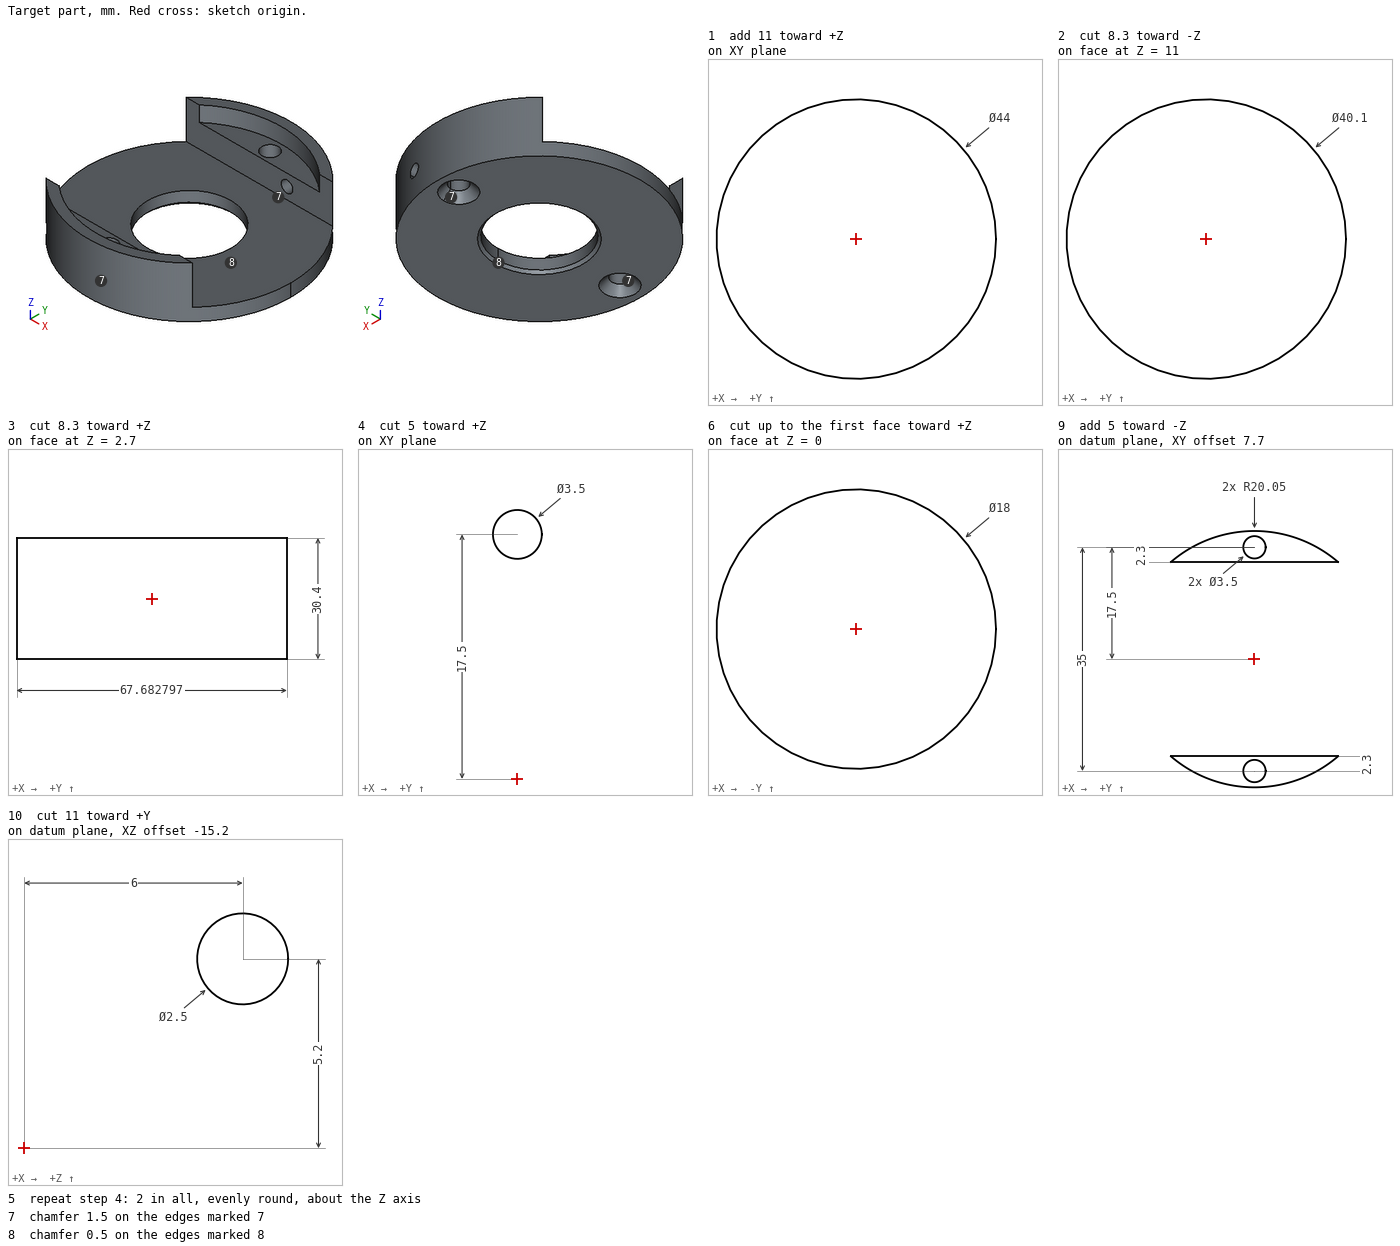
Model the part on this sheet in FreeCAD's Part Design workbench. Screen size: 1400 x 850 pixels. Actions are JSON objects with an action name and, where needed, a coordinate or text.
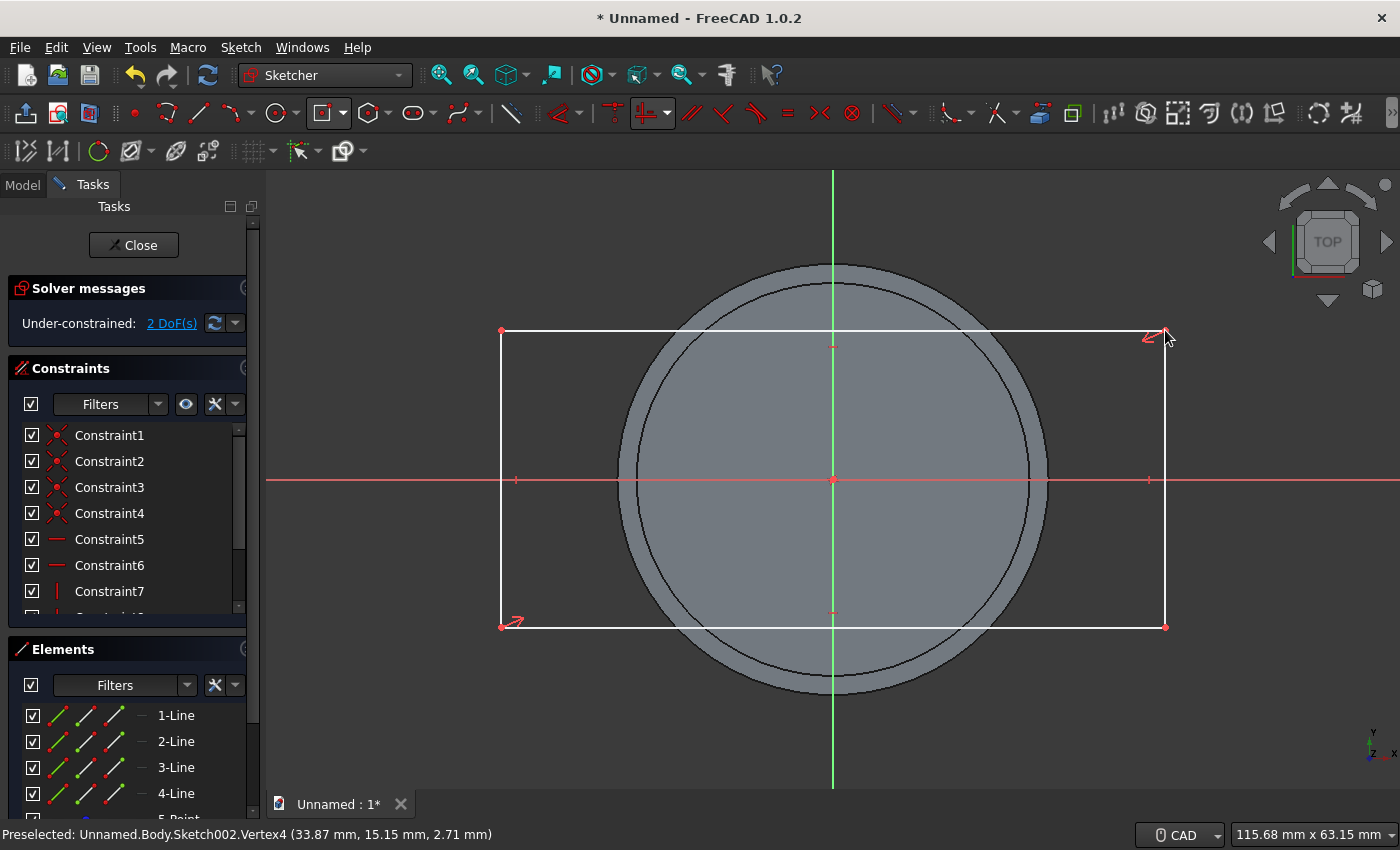
{"action": "left_click", "coordinate": [558, 114]}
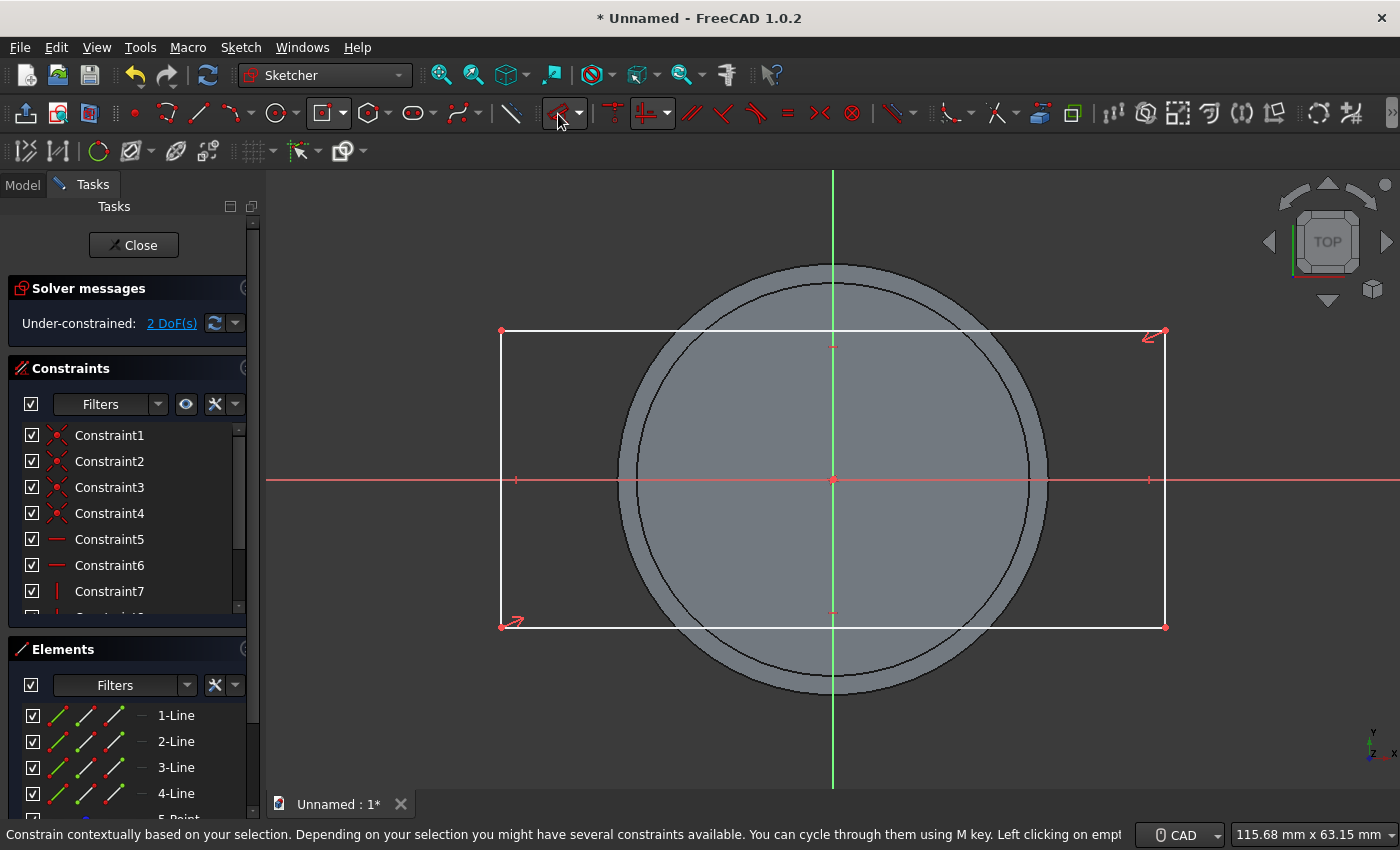
{"action": "left_click", "coordinate": [1165, 539]}
{"action": "left_click", "coordinate": [1199, 411]}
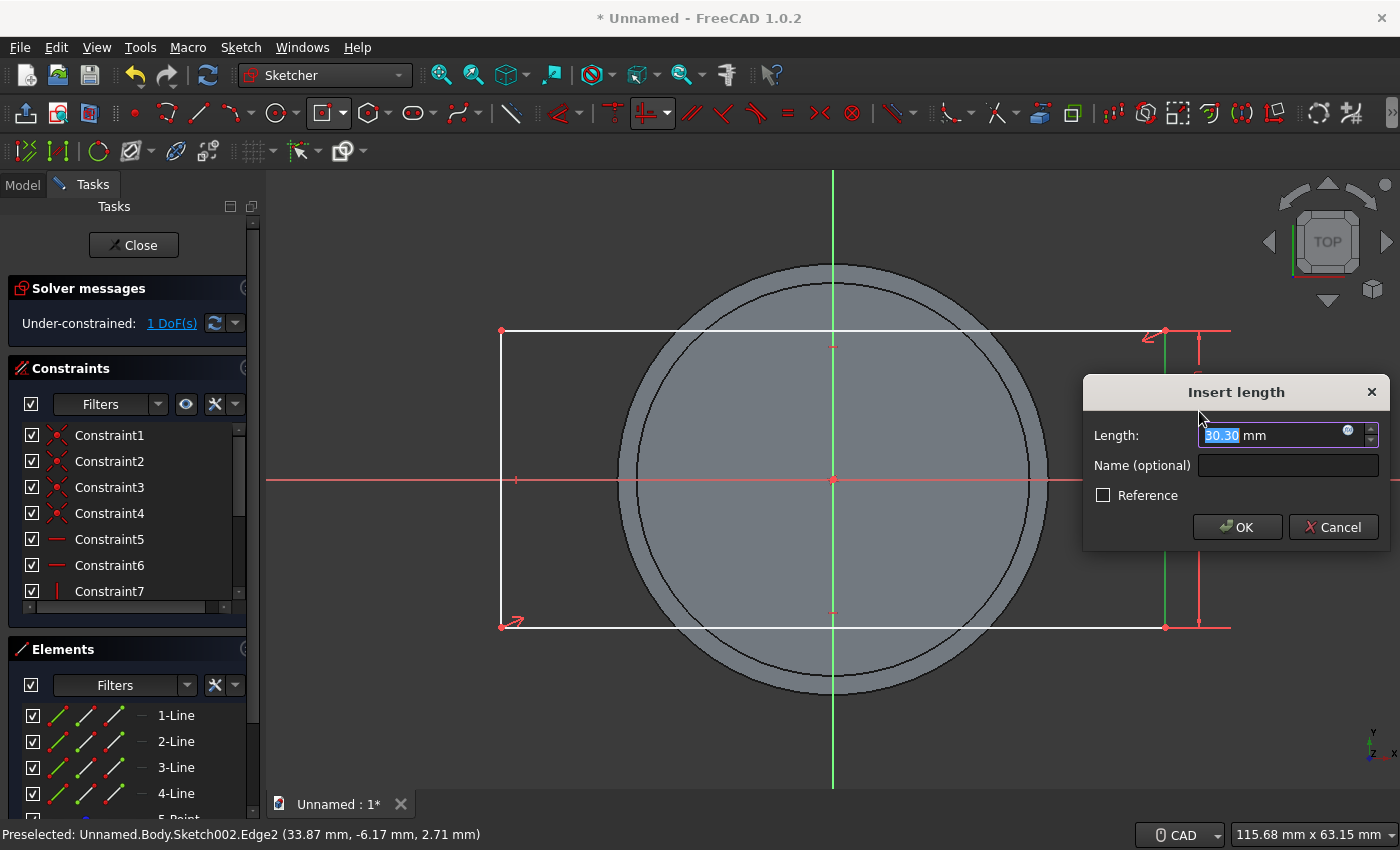
{"action": "type", "text": "30.4"}
{"action": "key", "text": "Return"}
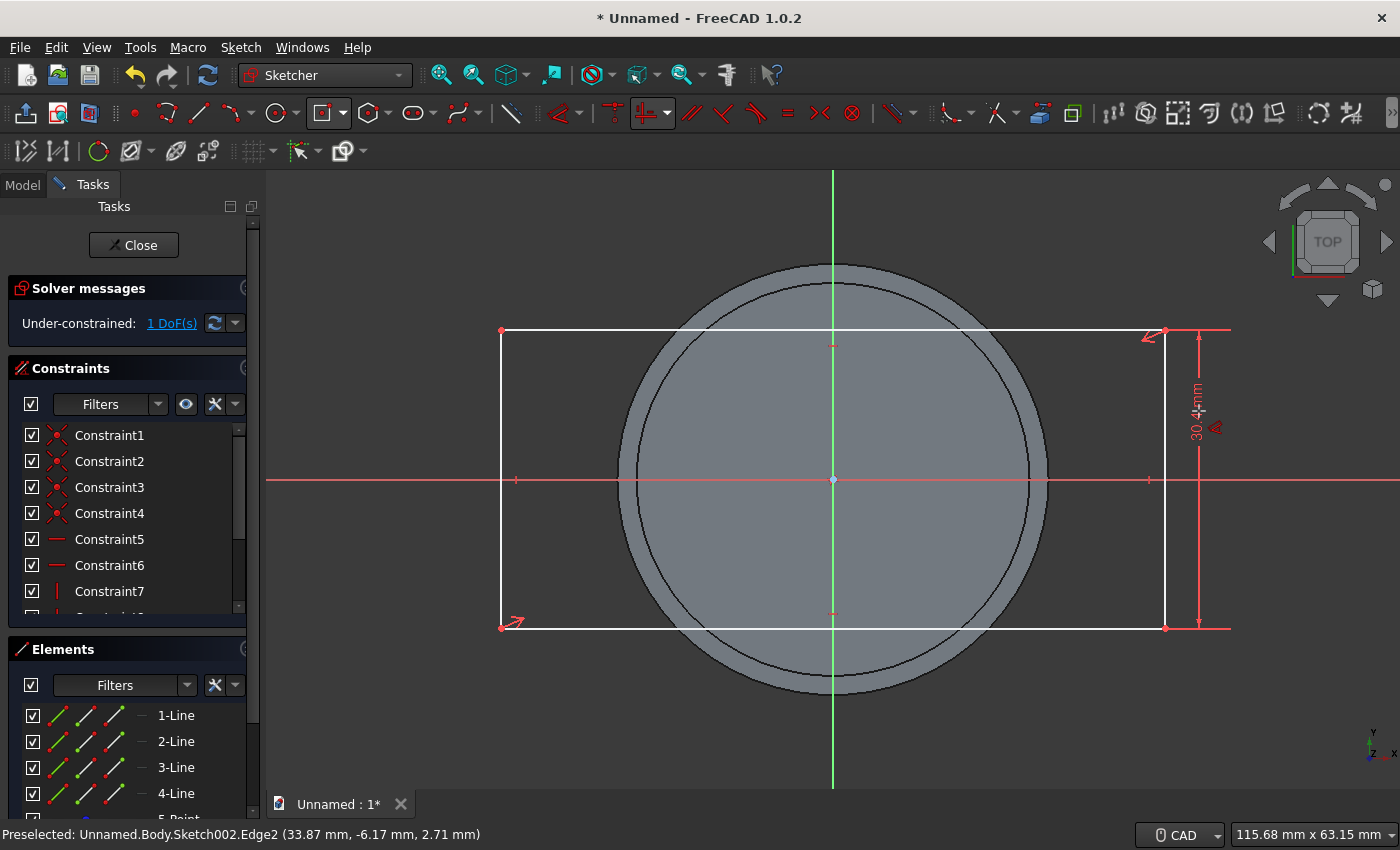
{"action": "left_click", "coordinate": [700, 629]}
{"action": "left_click", "coordinate": [680, 663]}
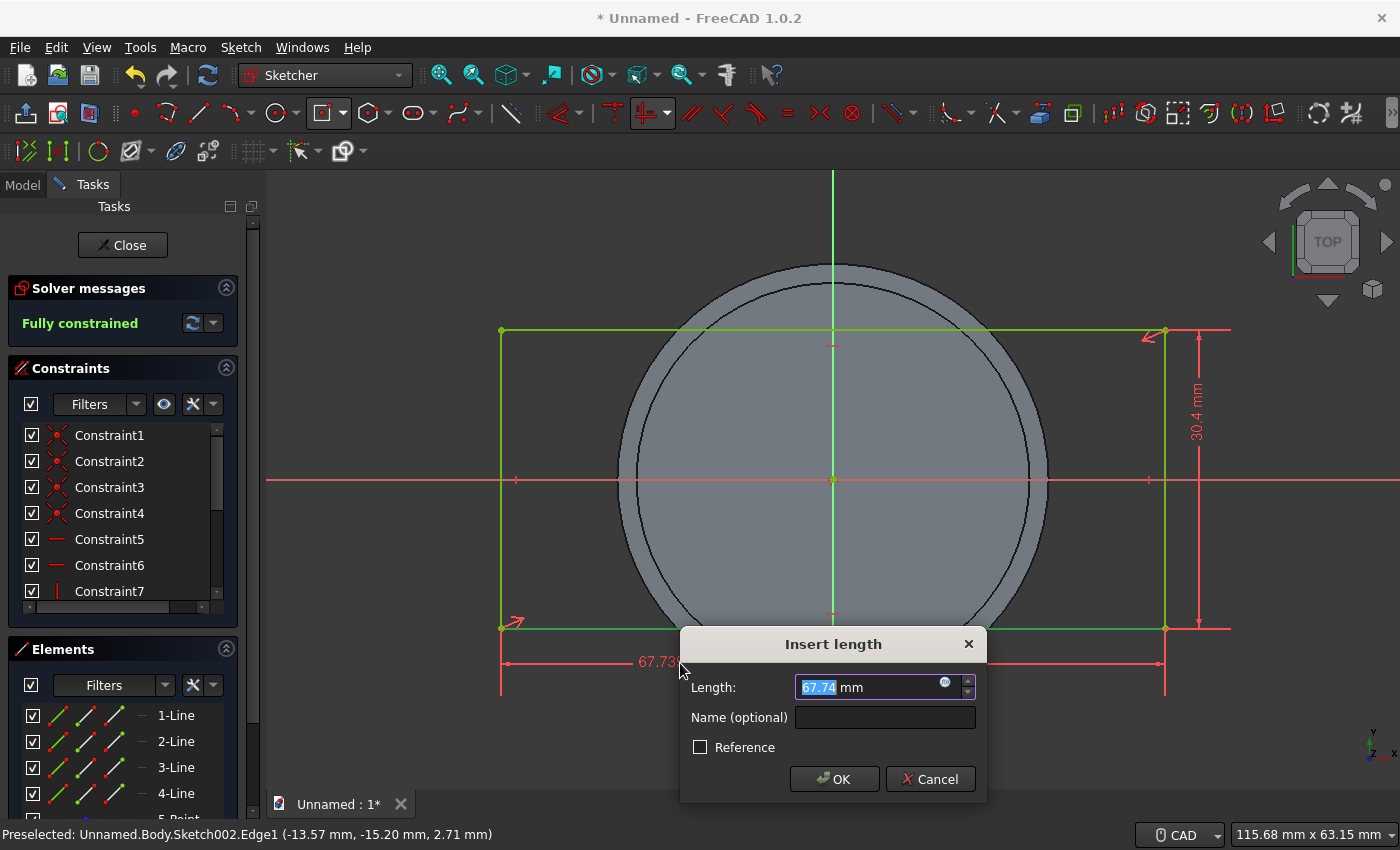
{"action": "type", "text": "67.682797"}
{"action": "key", "text": "Return"}
{"action": "key", "text": "Escape"}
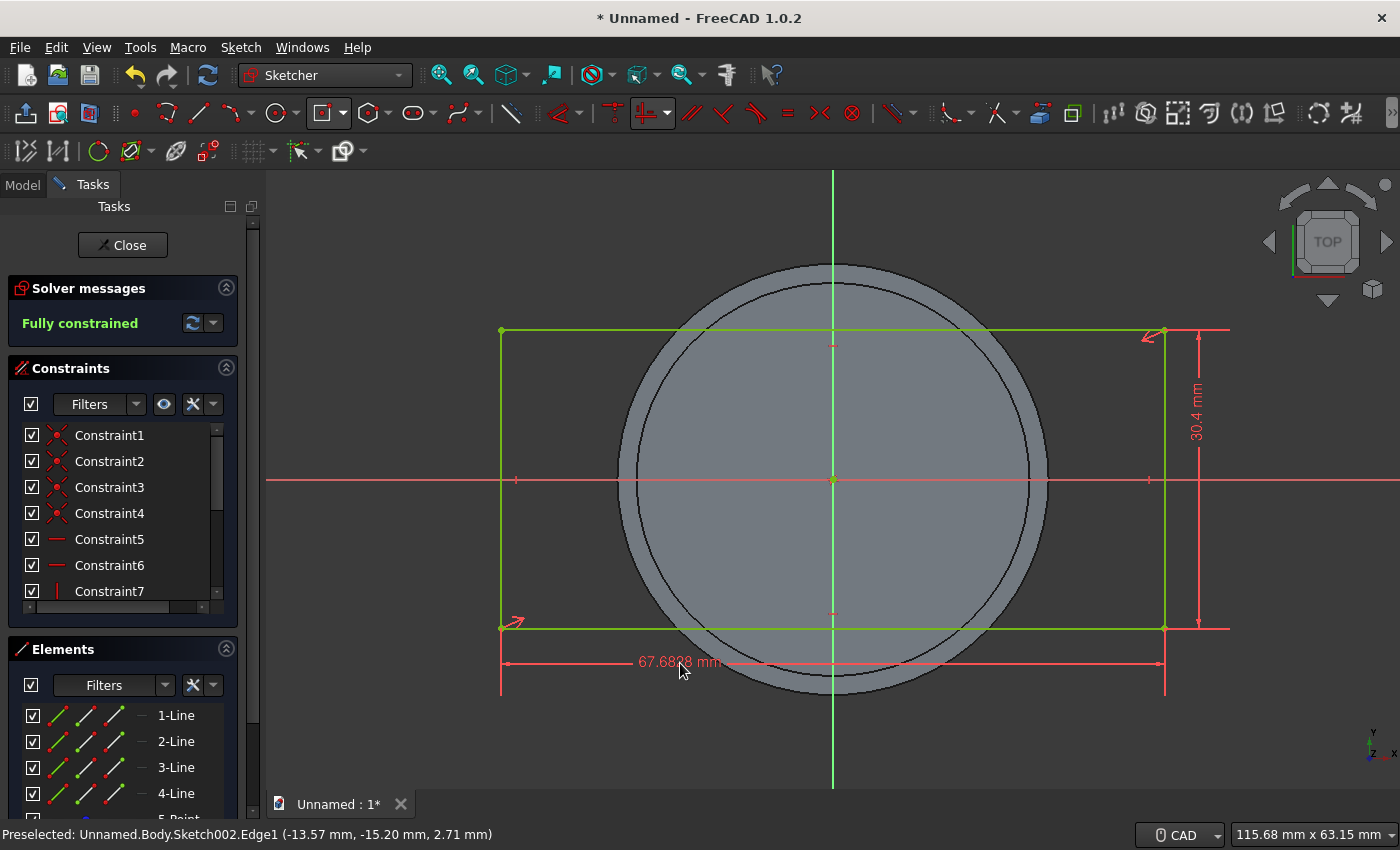
{"action": "left_click", "coordinate": [123, 245]}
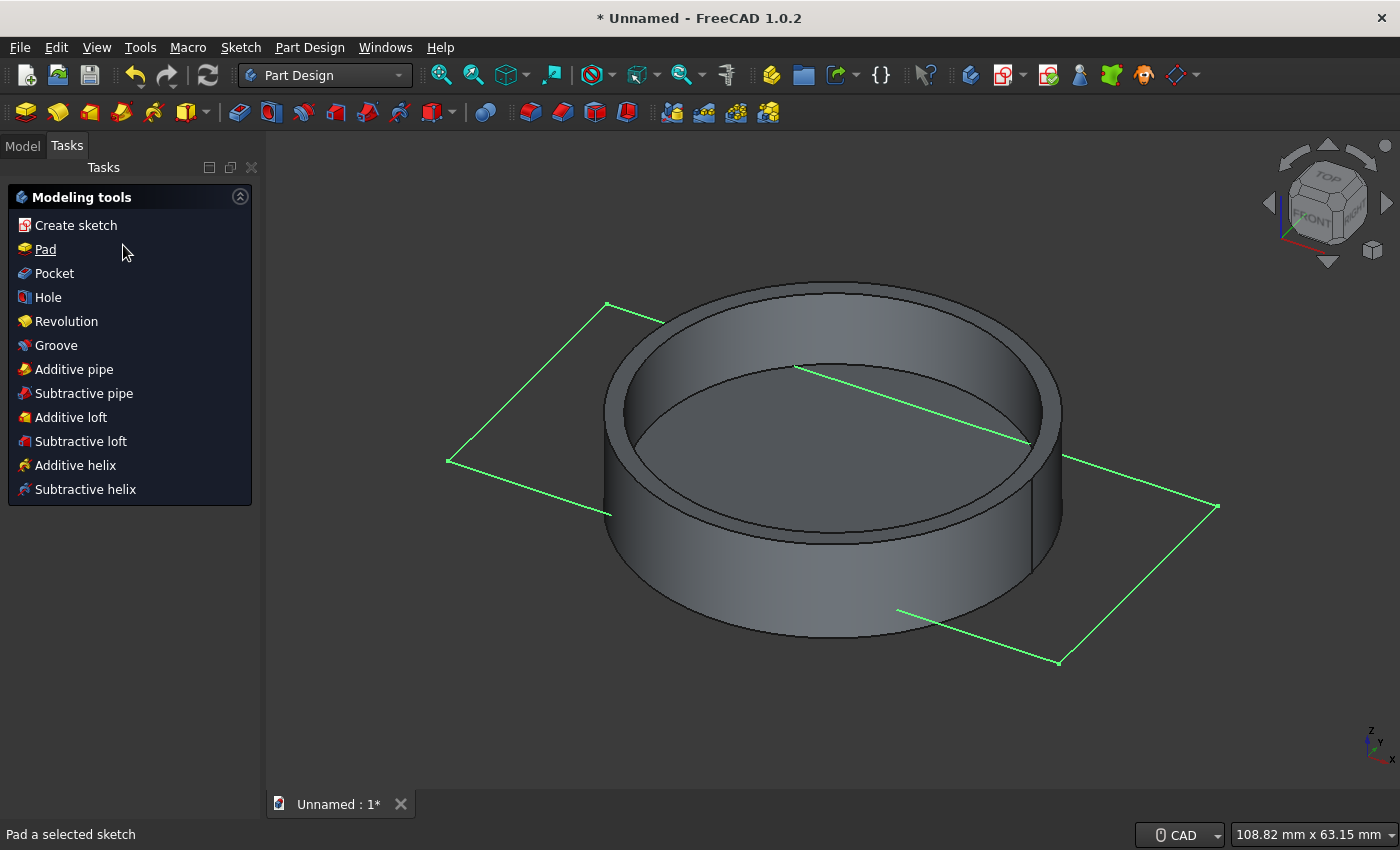
{"action": "left_click", "coordinate": [240, 112]}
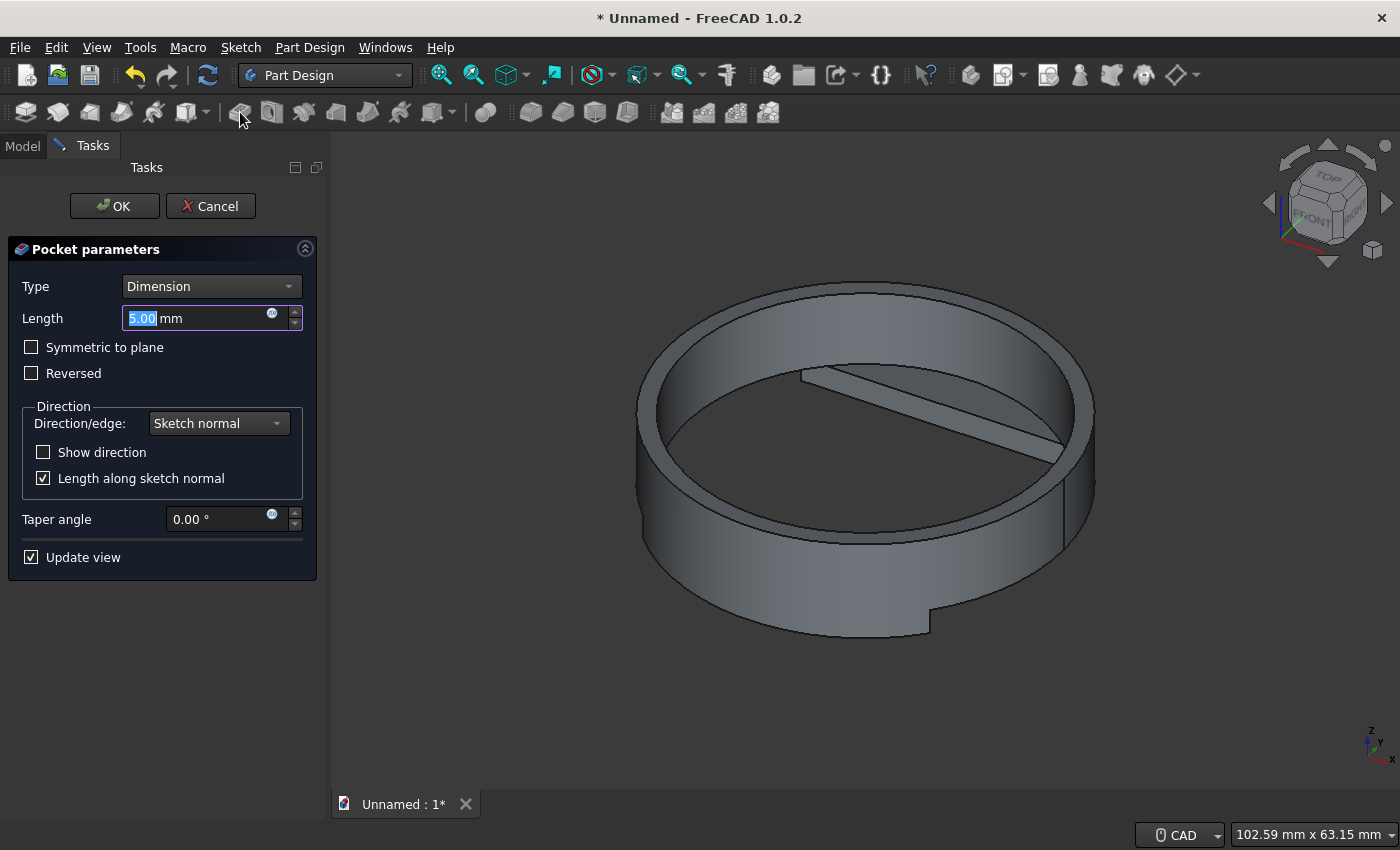
{"action": "type", "text": "8.3"}
{"action": "key", "text": "Tab"}